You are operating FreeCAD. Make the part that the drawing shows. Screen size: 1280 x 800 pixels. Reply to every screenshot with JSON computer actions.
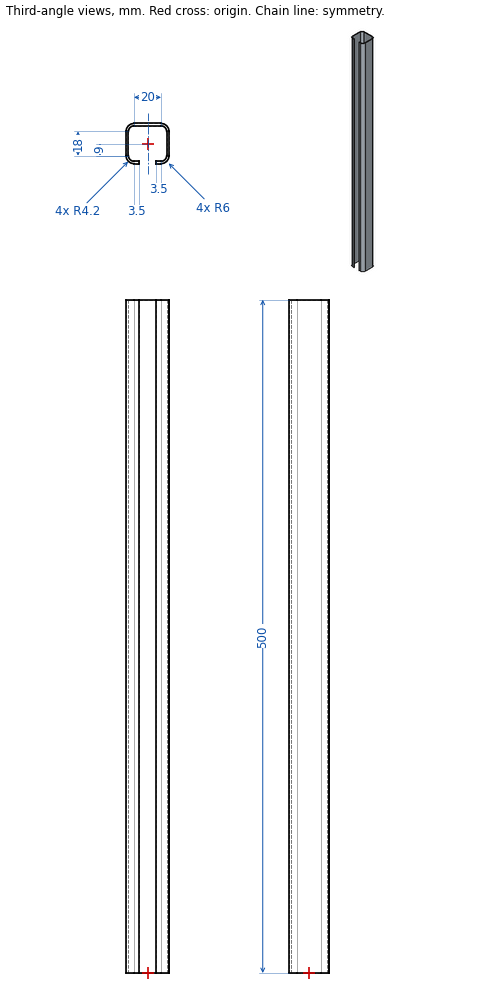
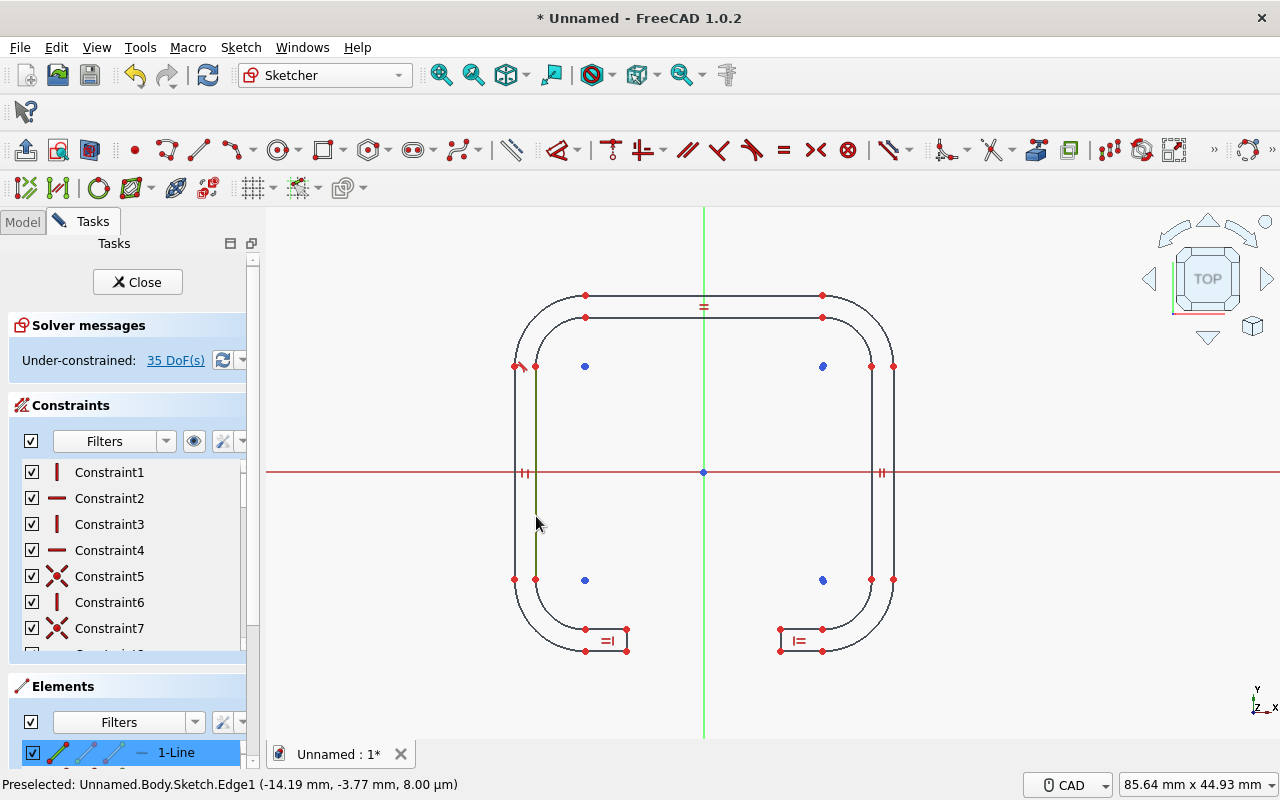
{"action": "left_click", "coordinate": [541, 602]}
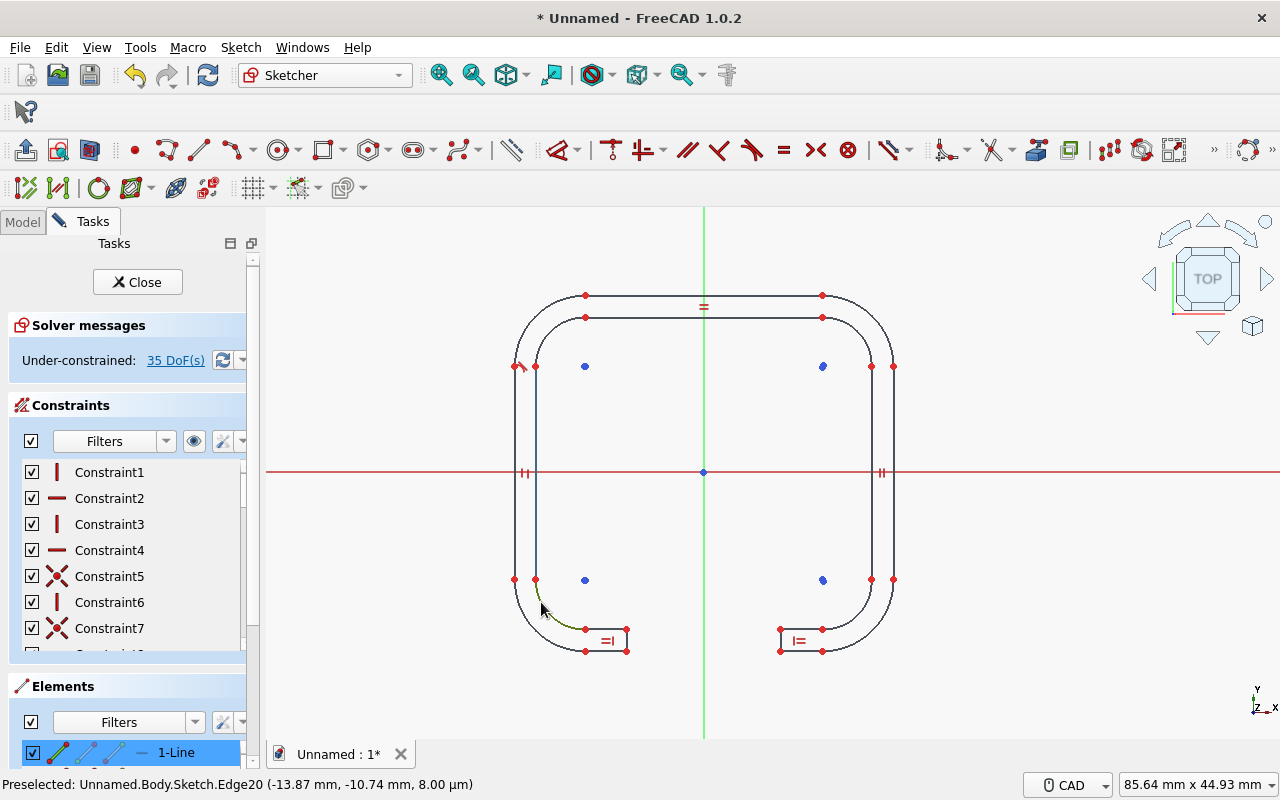
{"action": "left_click", "coordinate": [752, 150]}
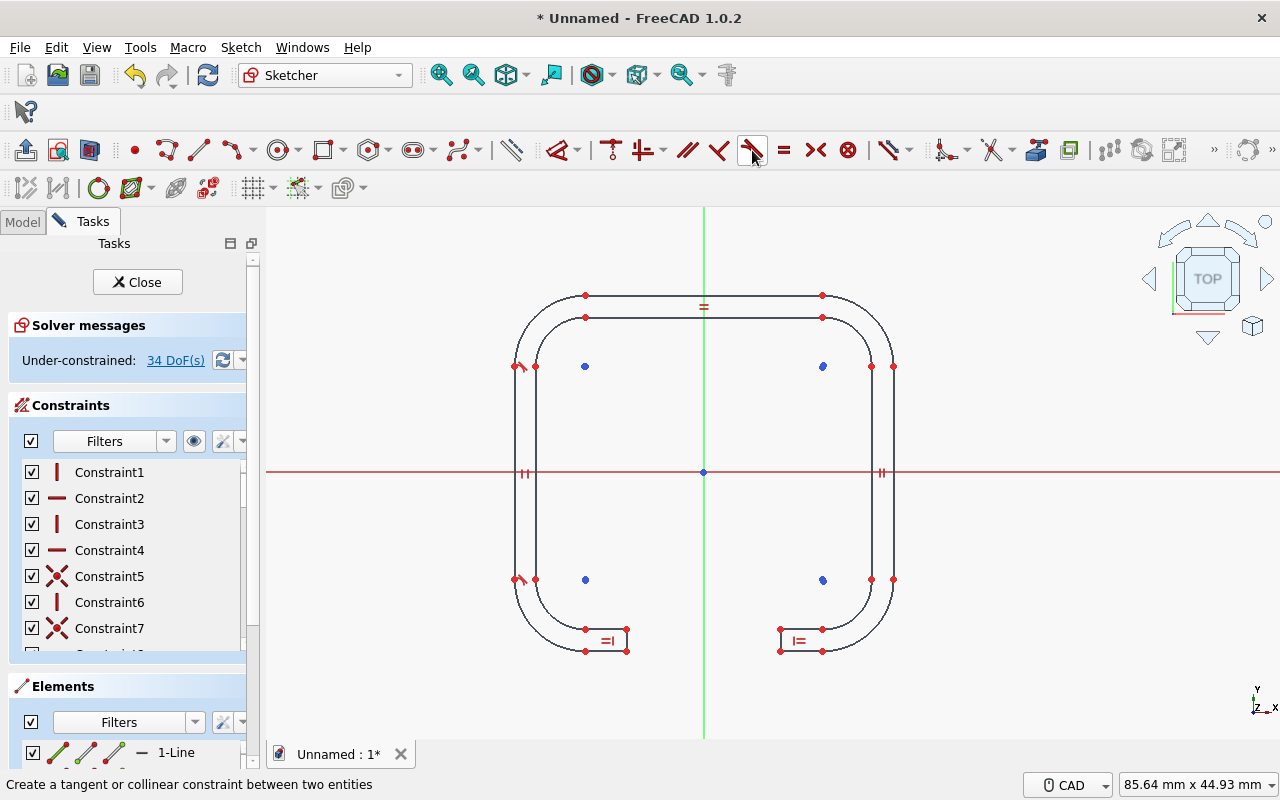
{"action": "left_click", "coordinate": [657, 318]}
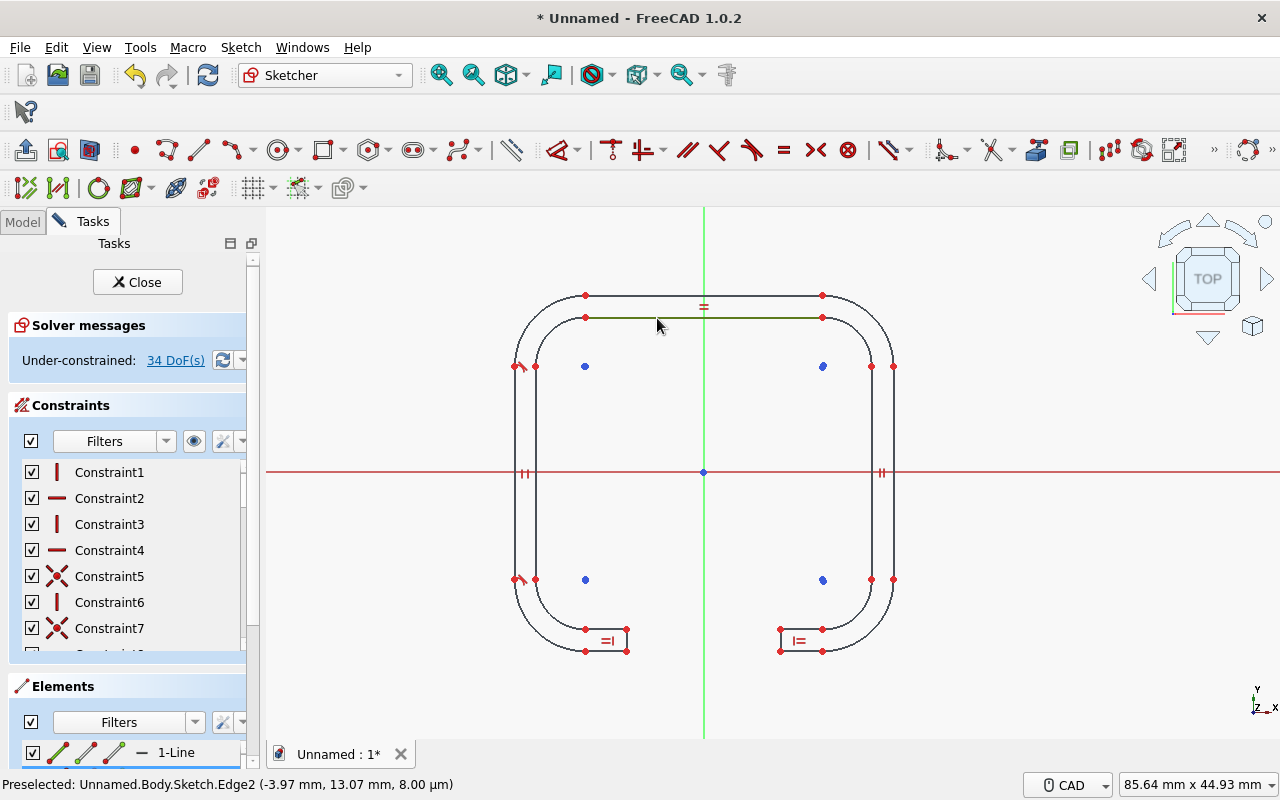
{"action": "left_click", "coordinate": [563, 323]}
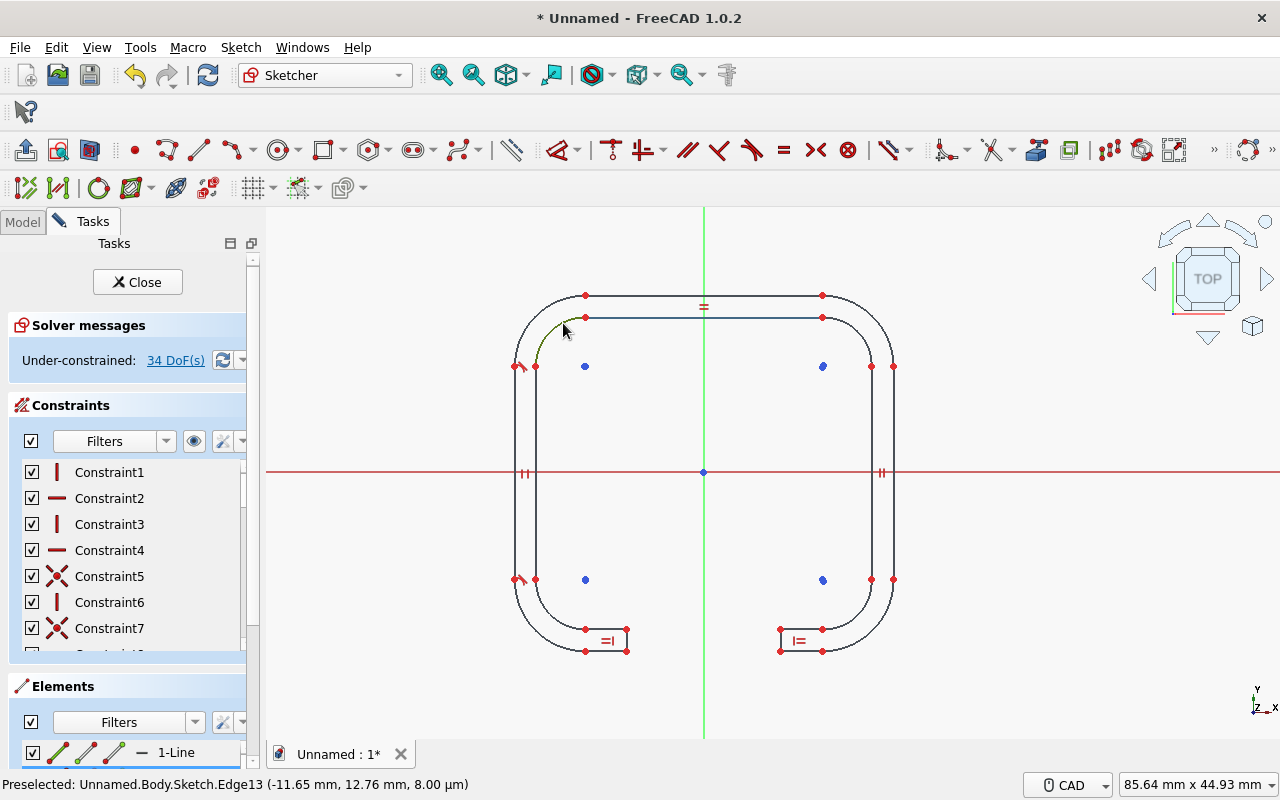
{"action": "left_click", "coordinate": [752, 150]}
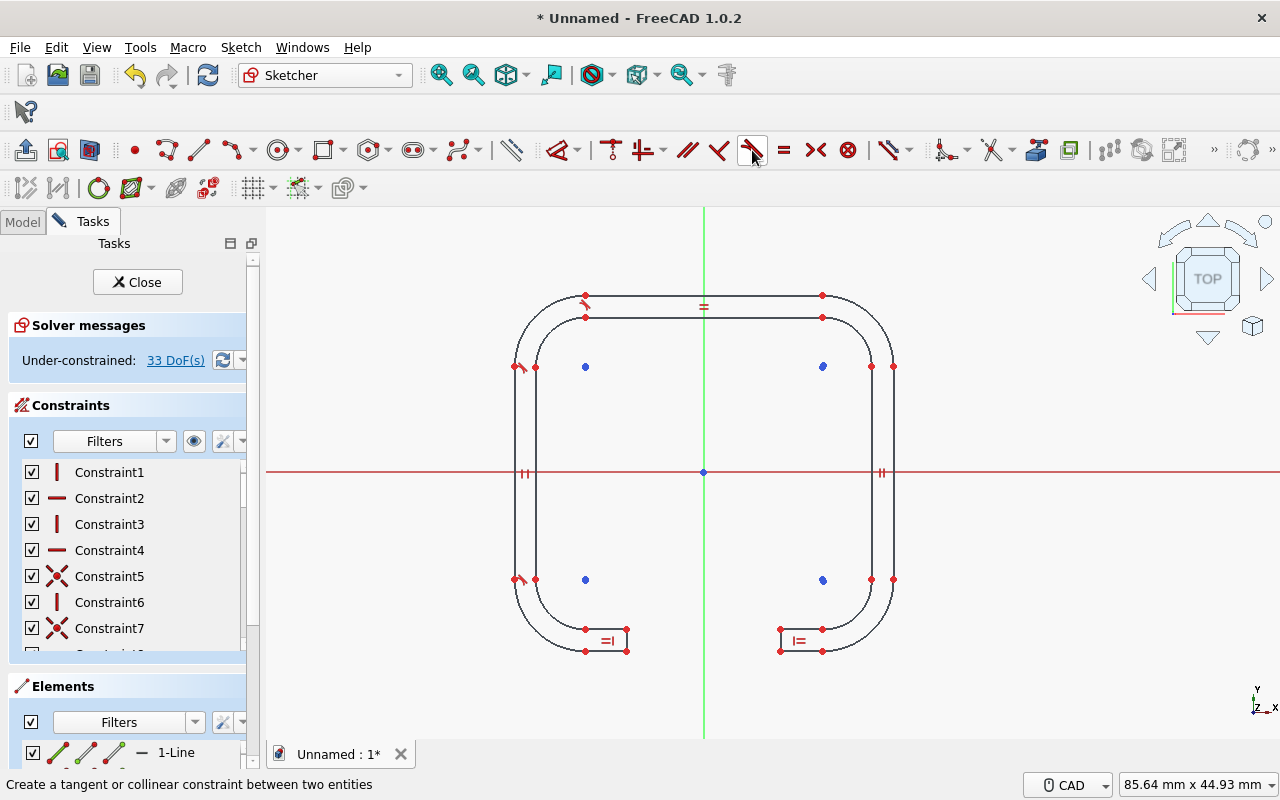
{"action": "left_click", "coordinate": [657, 318]}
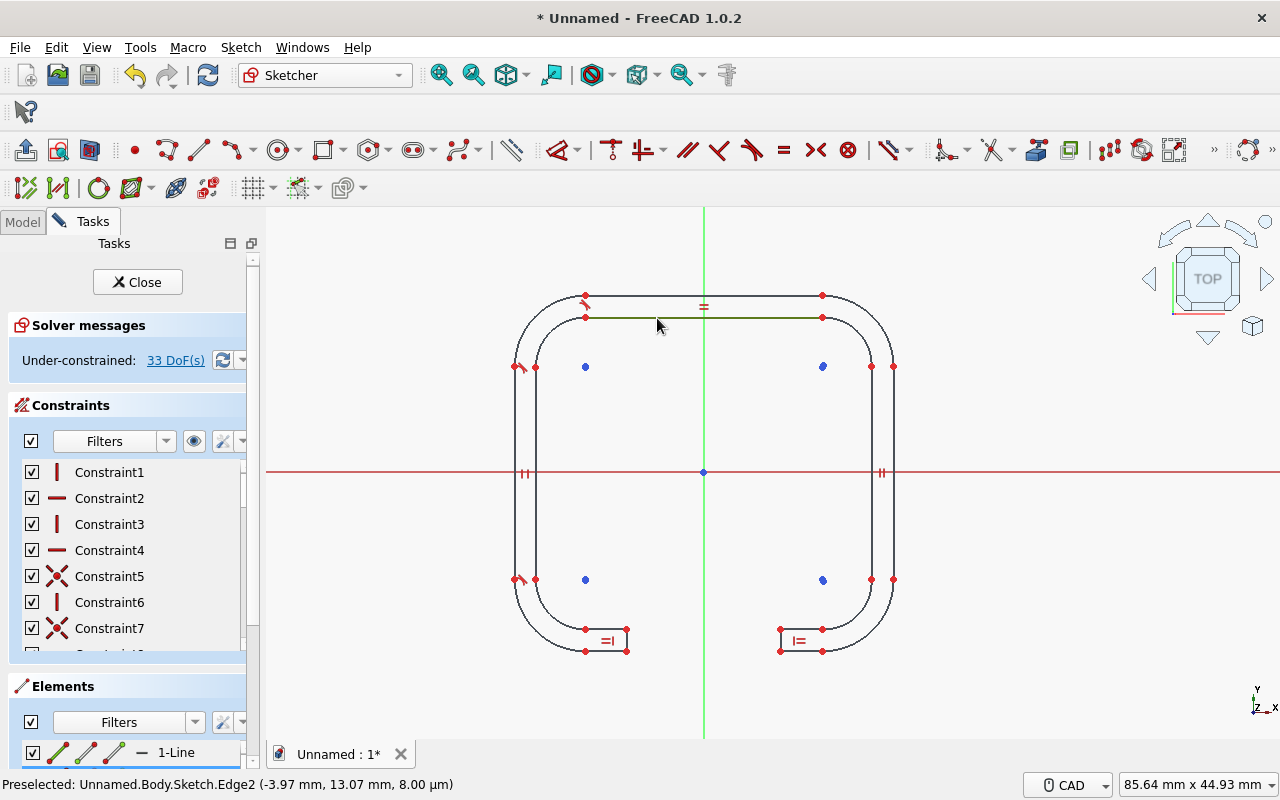
{"action": "left_click", "coordinate": [867, 344]}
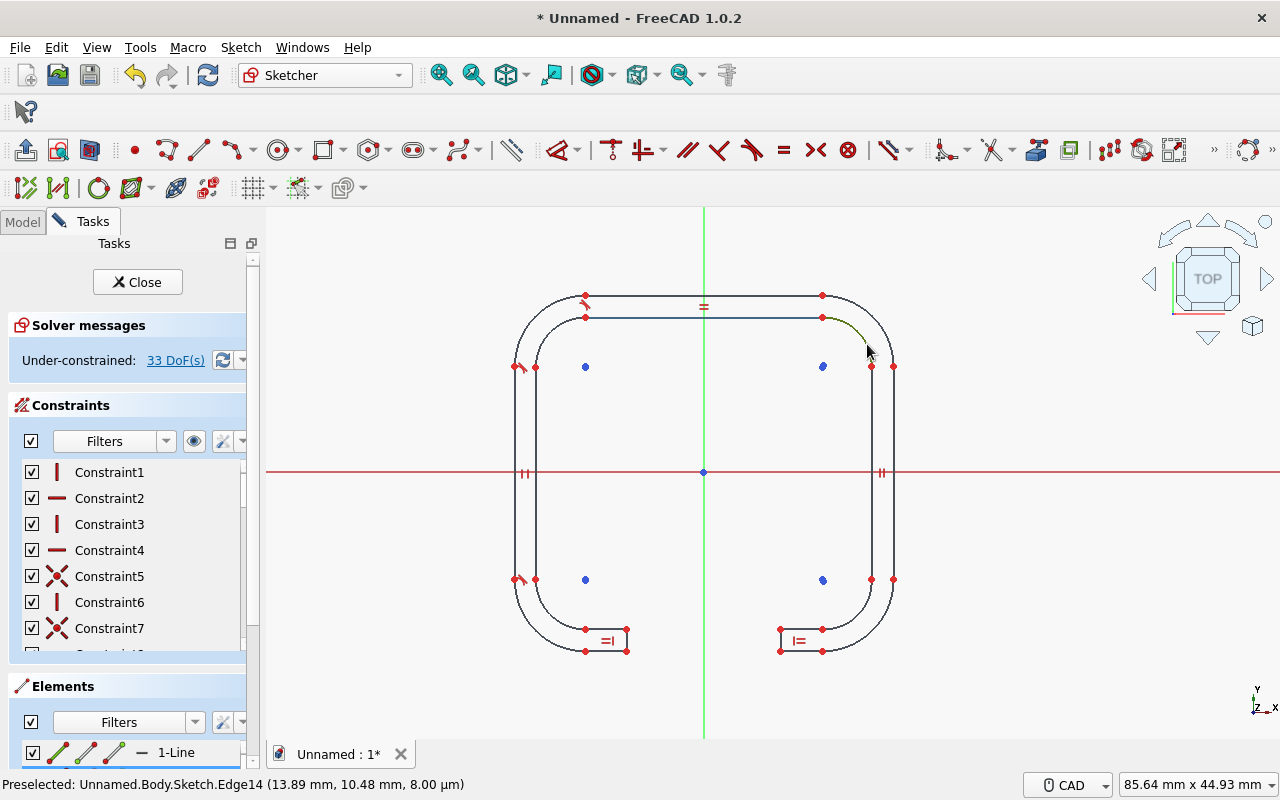
{"action": "left_click", "coordinate": [752, 150]}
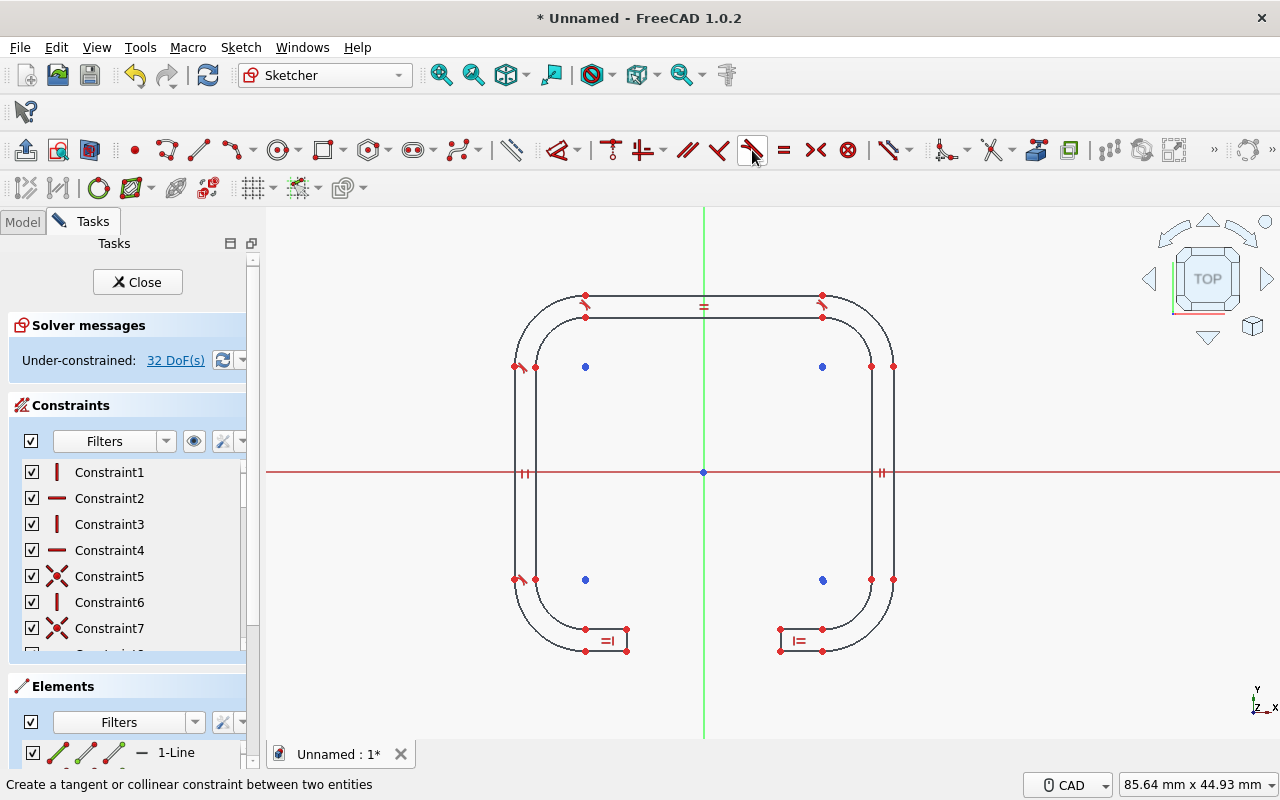
{"action": "left_click", "coordinate": [872, 430]}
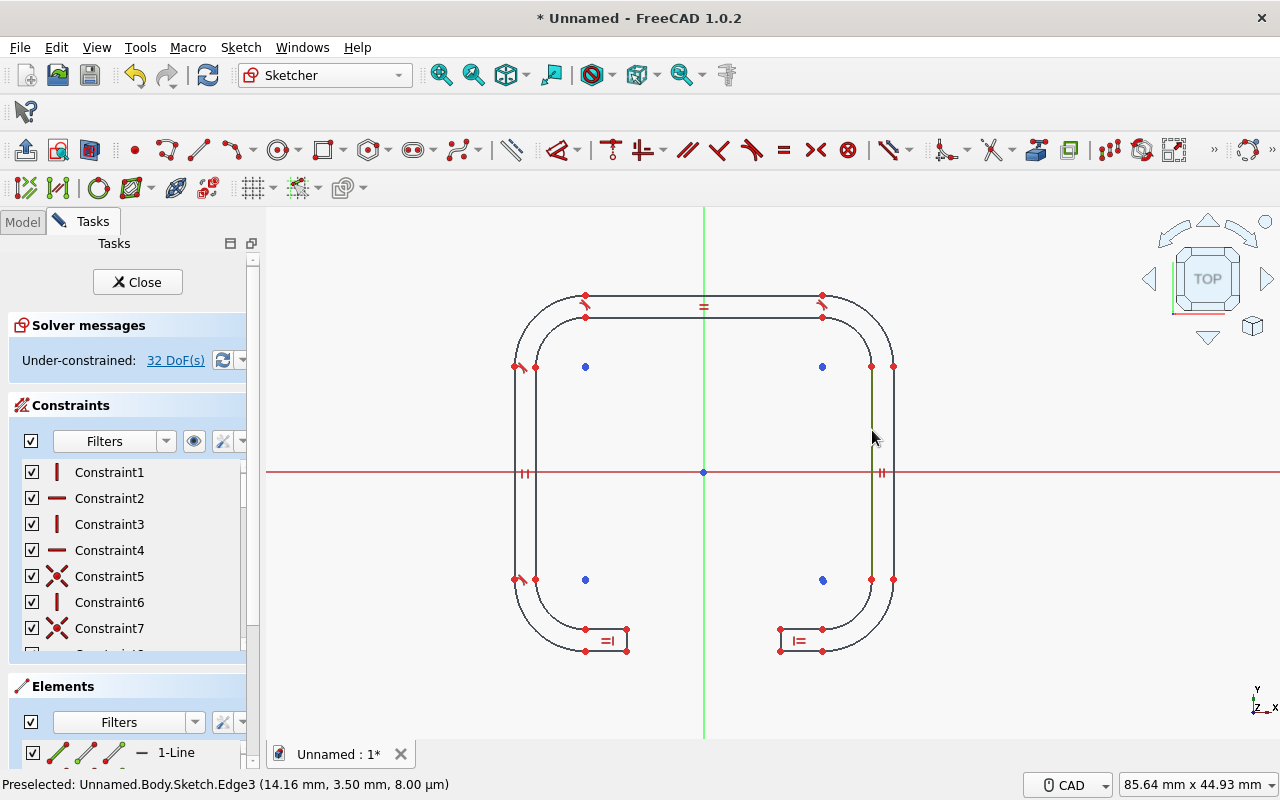
{"action": "left_click", "coordinate": [866, 344]}